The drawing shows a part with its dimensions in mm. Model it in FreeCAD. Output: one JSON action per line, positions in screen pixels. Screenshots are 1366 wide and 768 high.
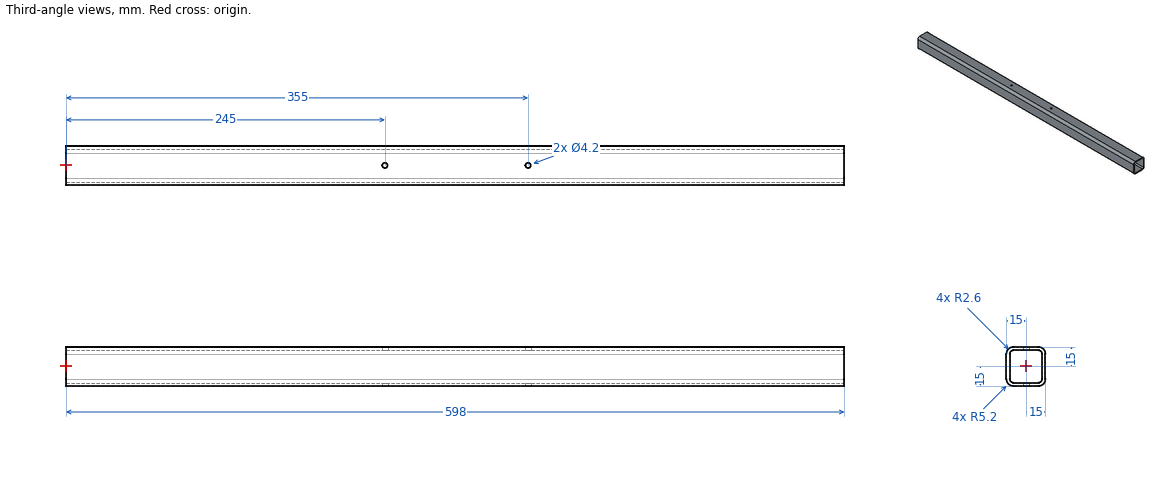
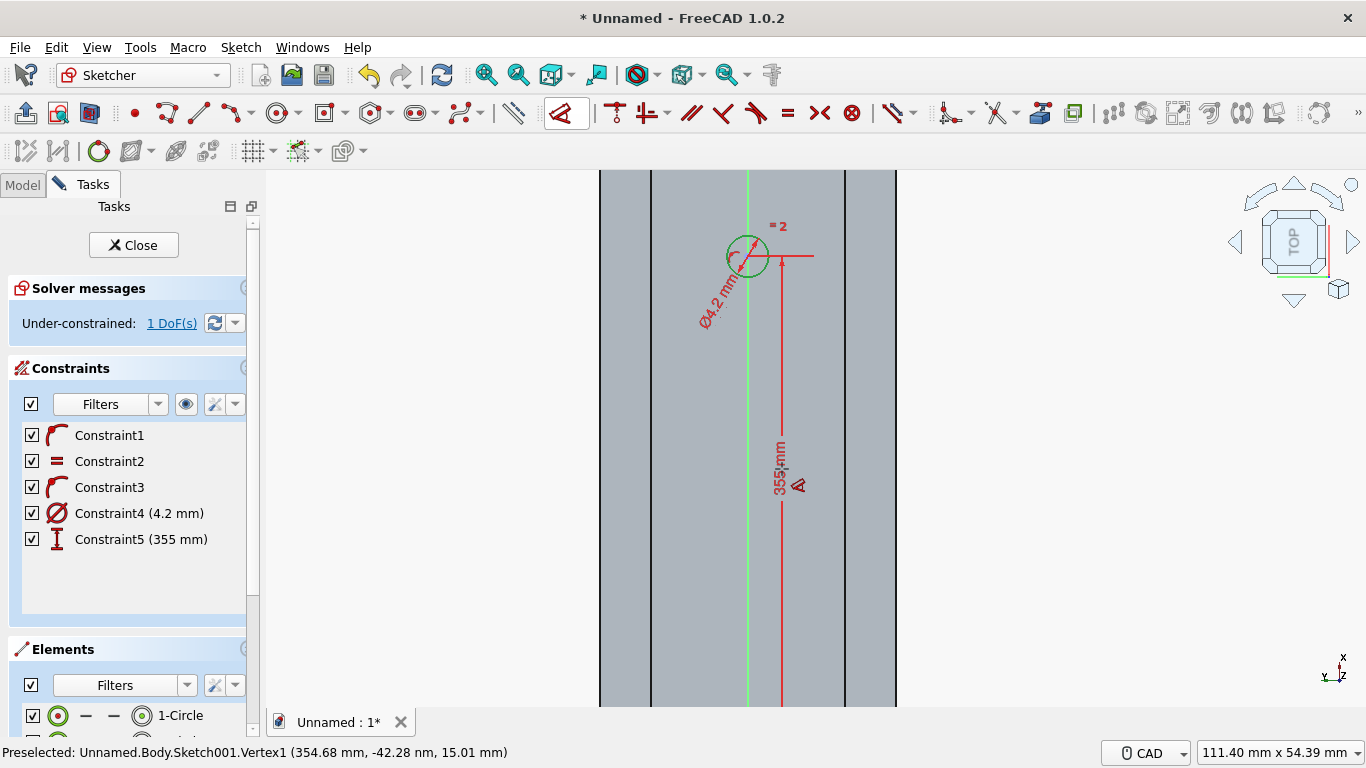
{"action": "scroll", "coordinate": [747, 283], "scroll_direction": "down", "scroll_amount": 6}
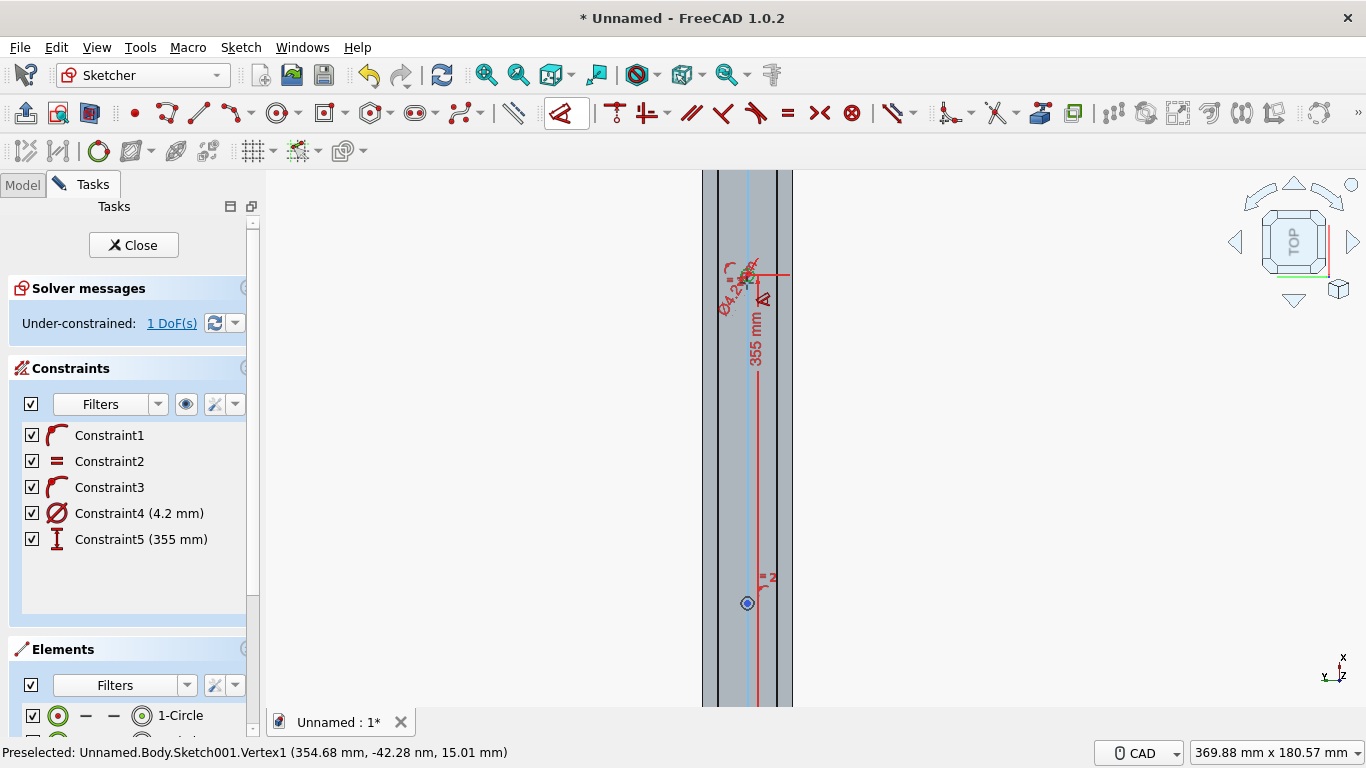
{"action": "left_click", "coordinate": [748, 603]}
{"action": "left_click", "coordinate": [782, 641]}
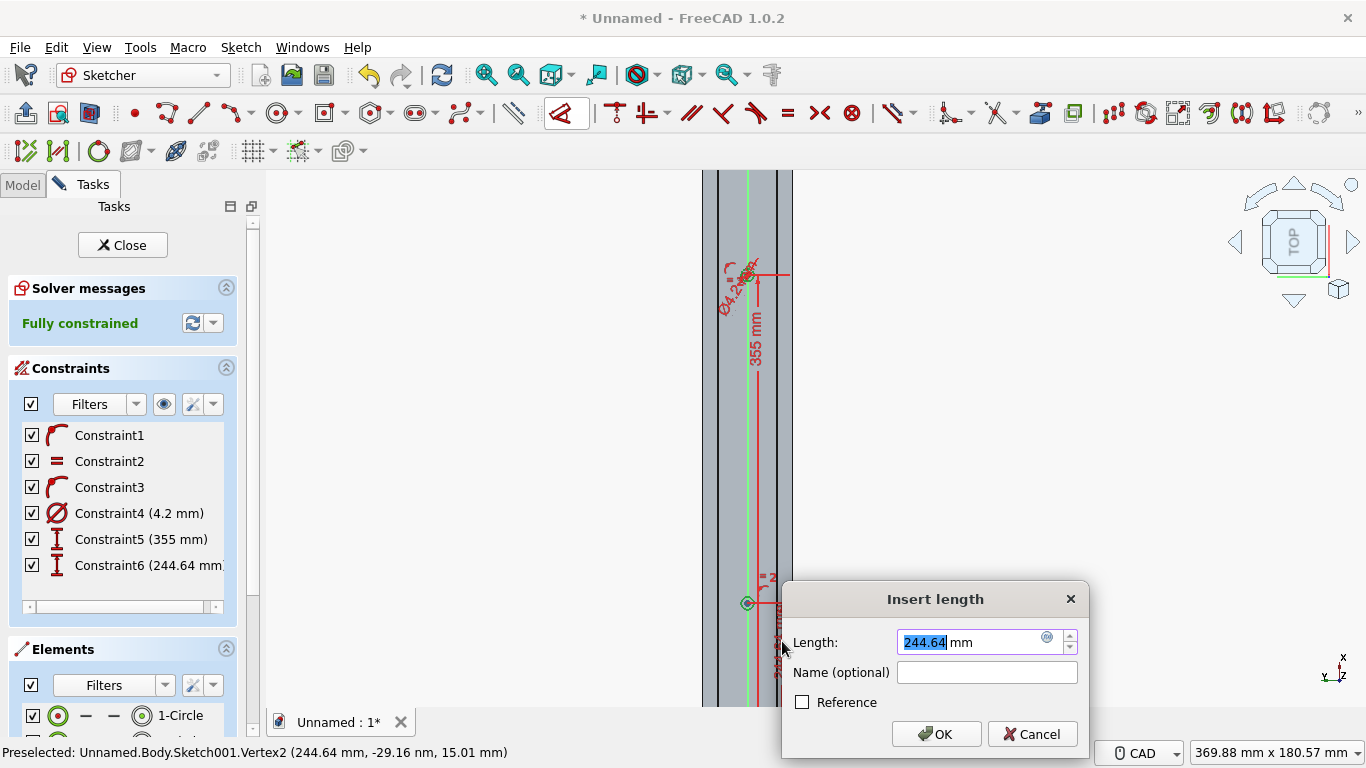
{"action": "type", "text": "245"}
{"action": "key", "text": "Return"}
{"action": "key", "text": "Escape"}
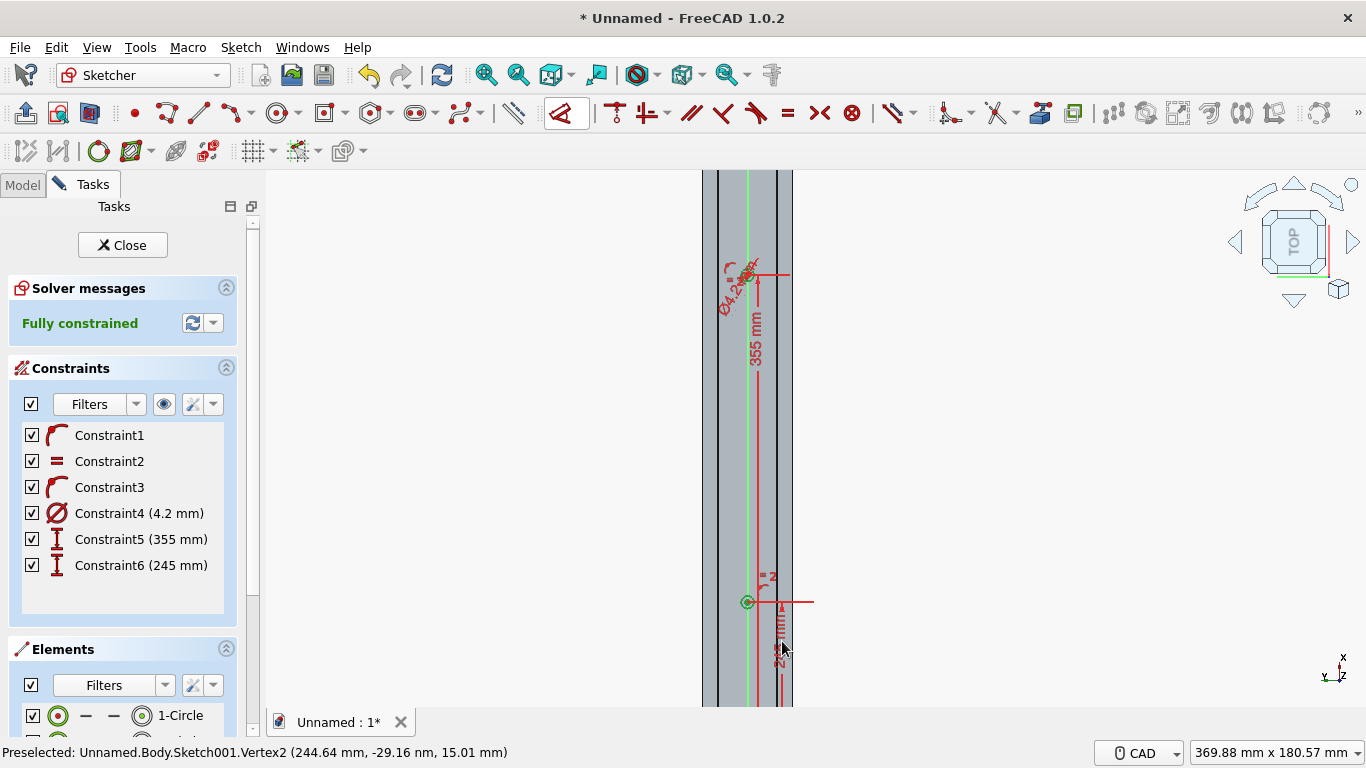
{"action": "left_click", "coordinate": [123, 245]}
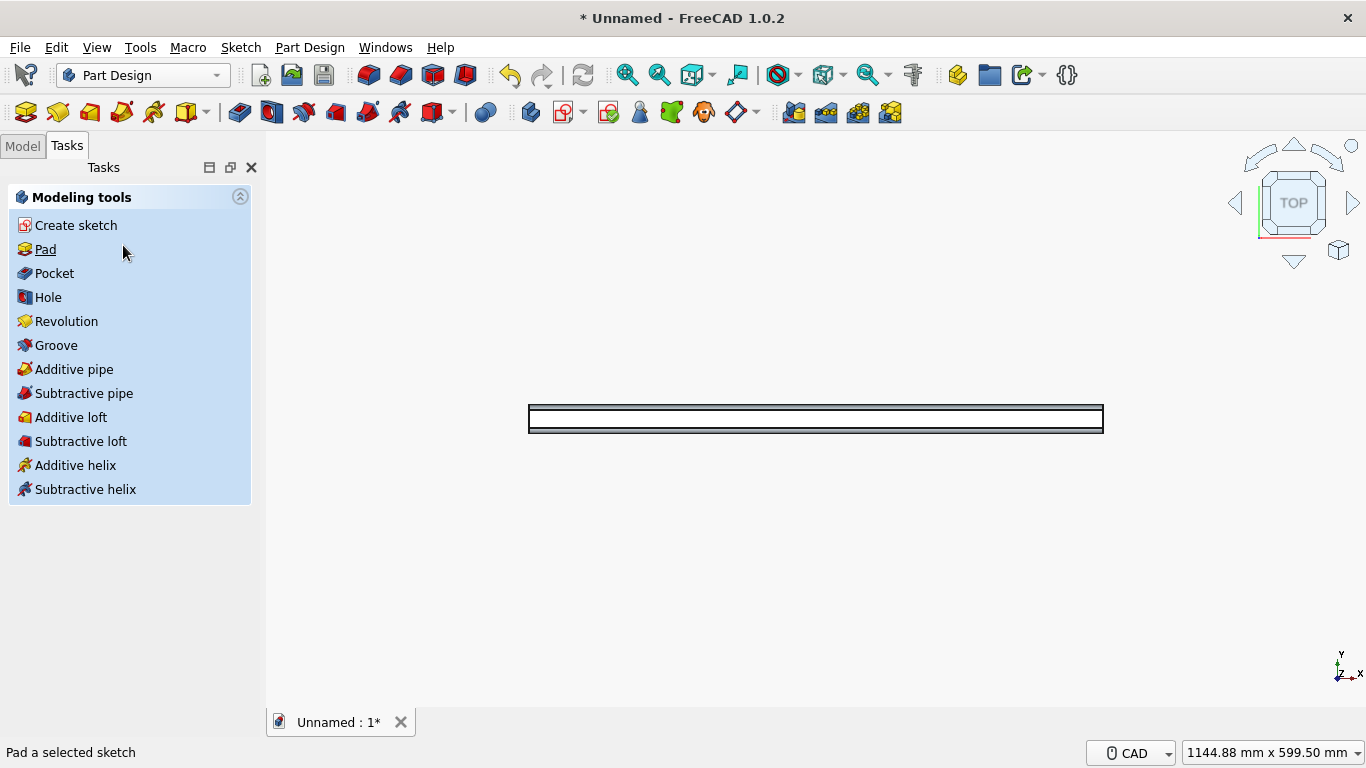
{"action": "left_click", "coordinate": [240, 112]}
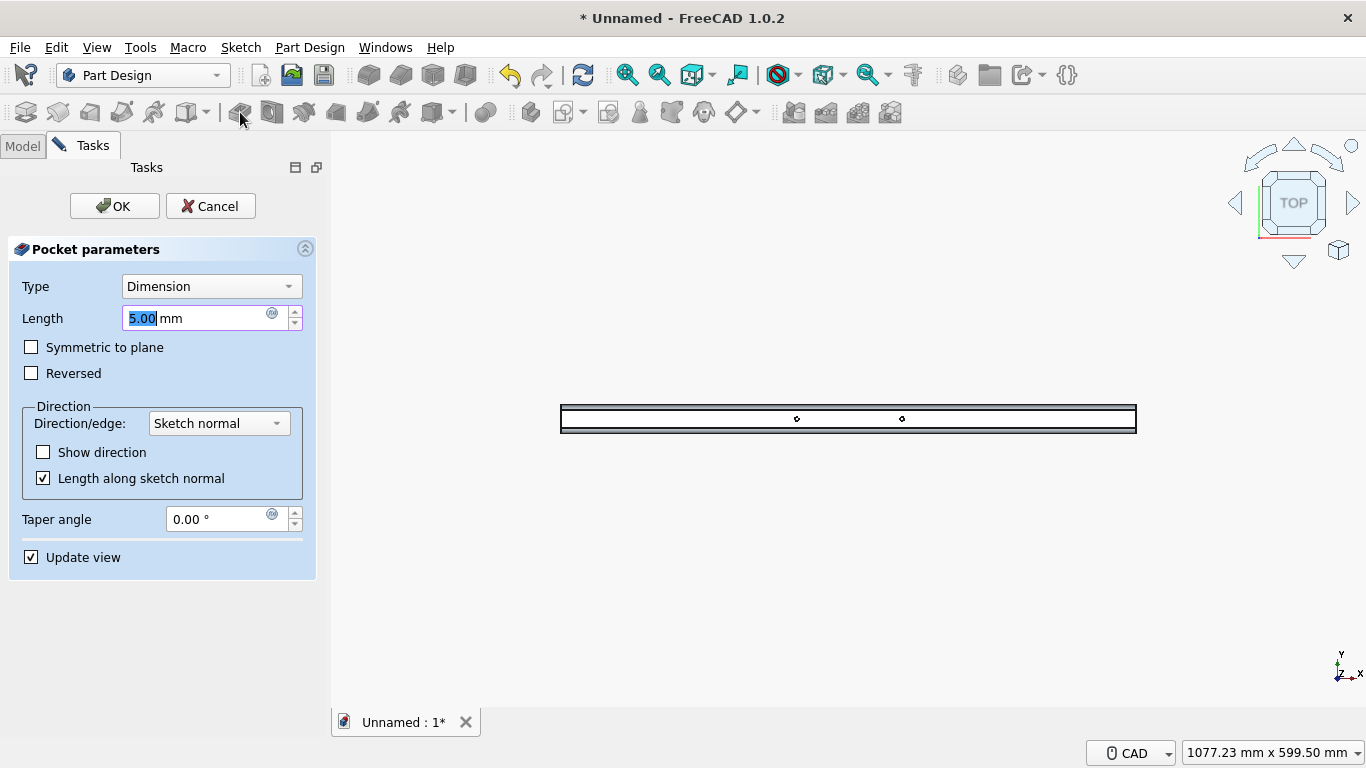
{"action": "left_click", "coordinate": [212, 286]}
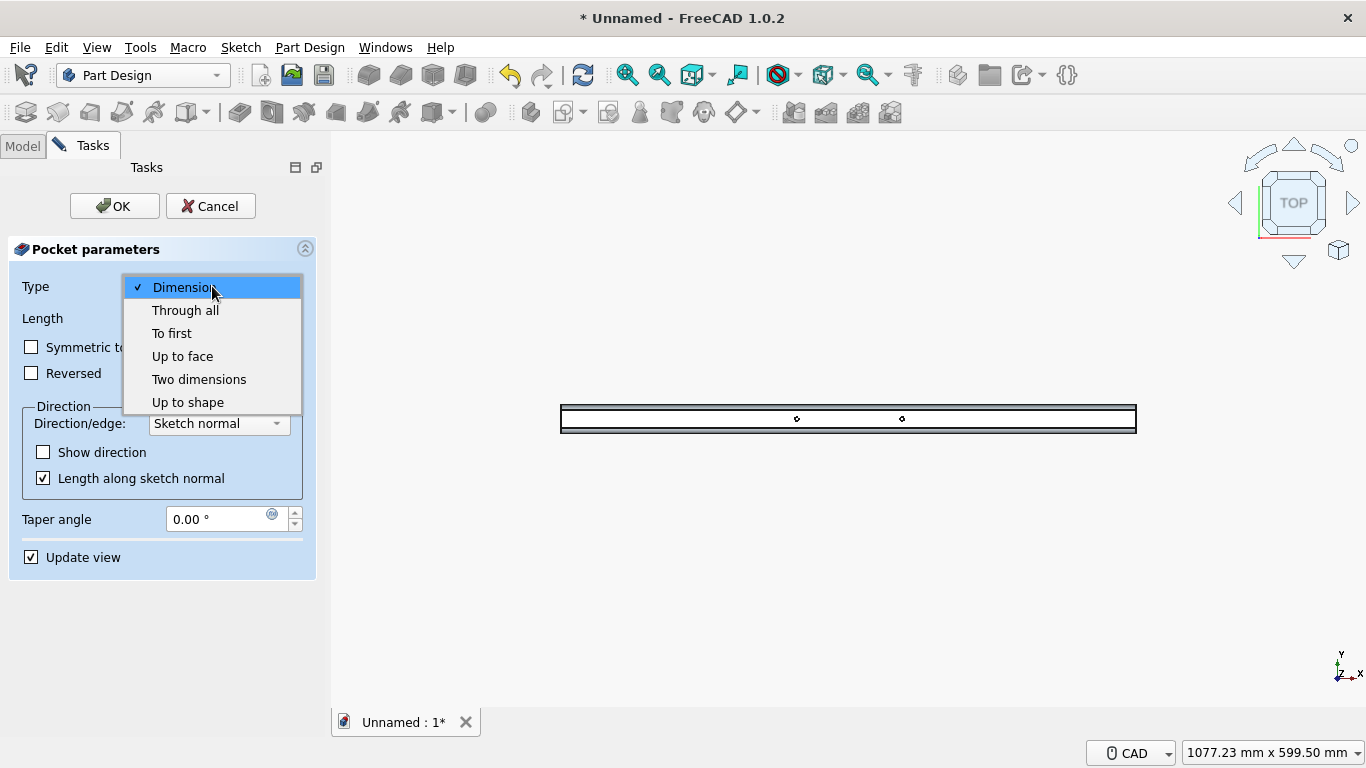
{"action": "left_click", "coordinate": [212, 310]}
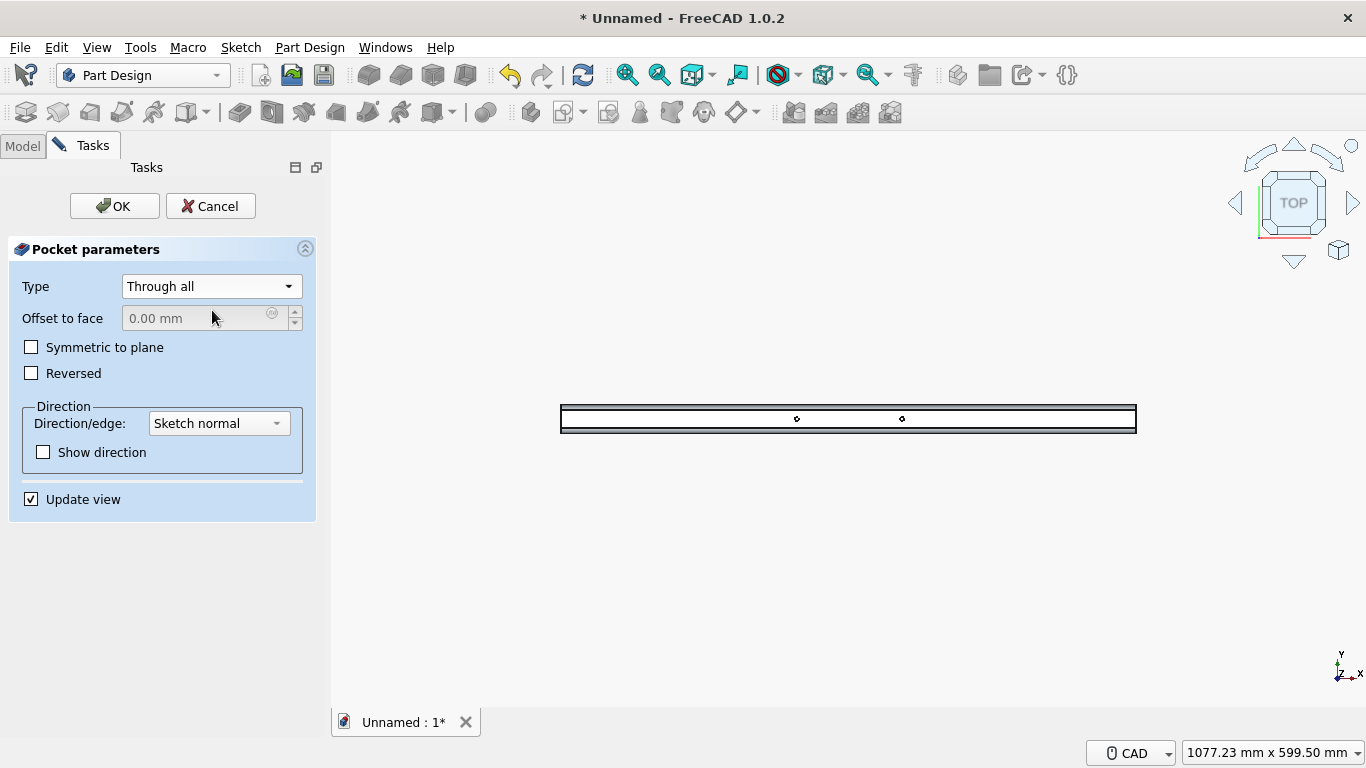
{"action": "left_click", "coordinate": [115, 206]}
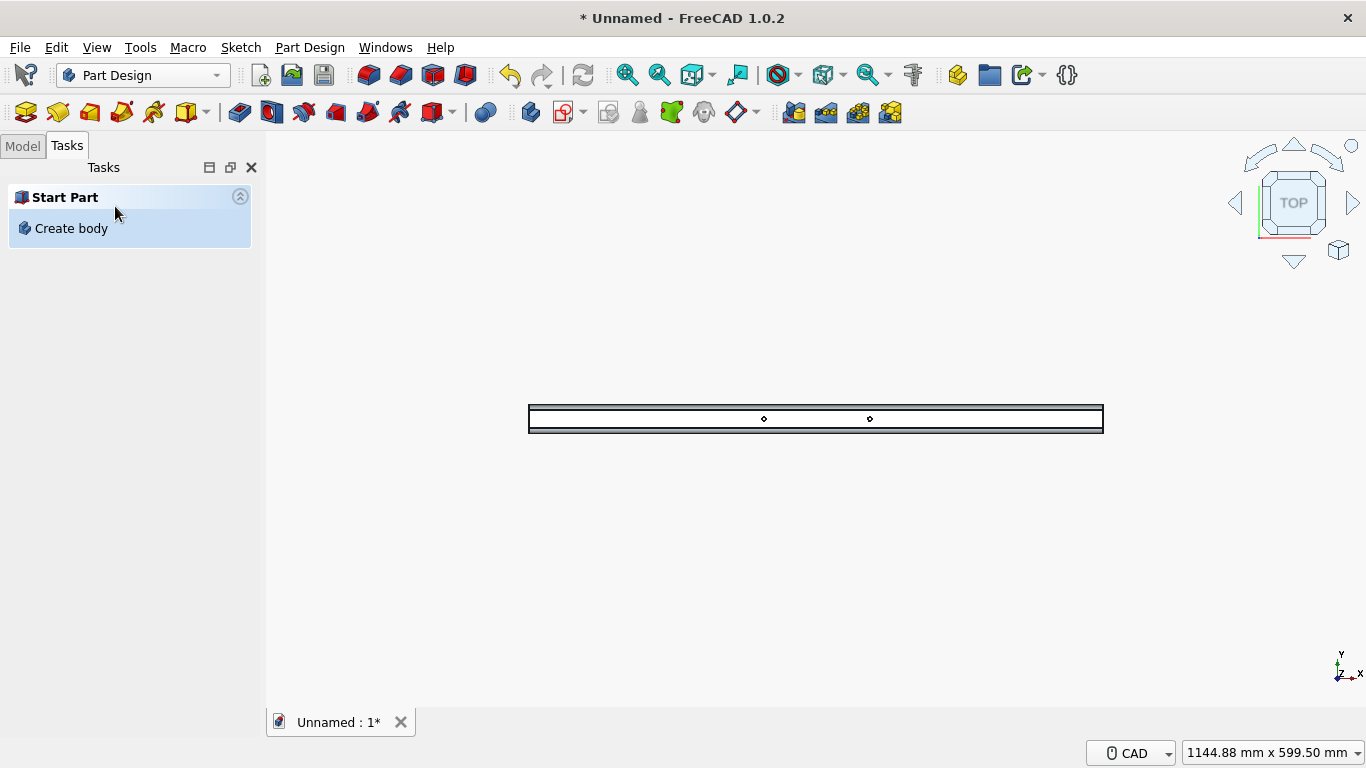
{"action": "key", "text": "0"}